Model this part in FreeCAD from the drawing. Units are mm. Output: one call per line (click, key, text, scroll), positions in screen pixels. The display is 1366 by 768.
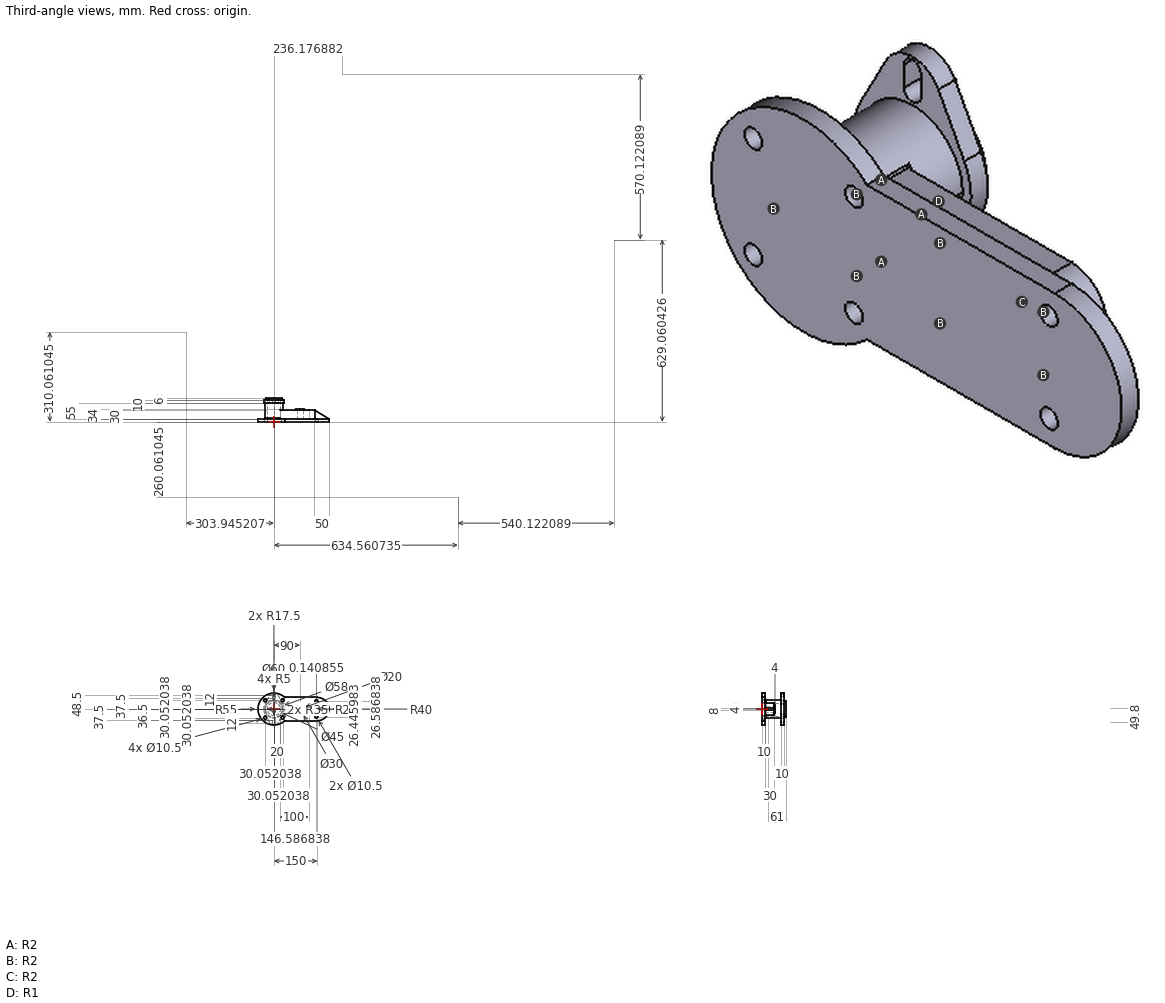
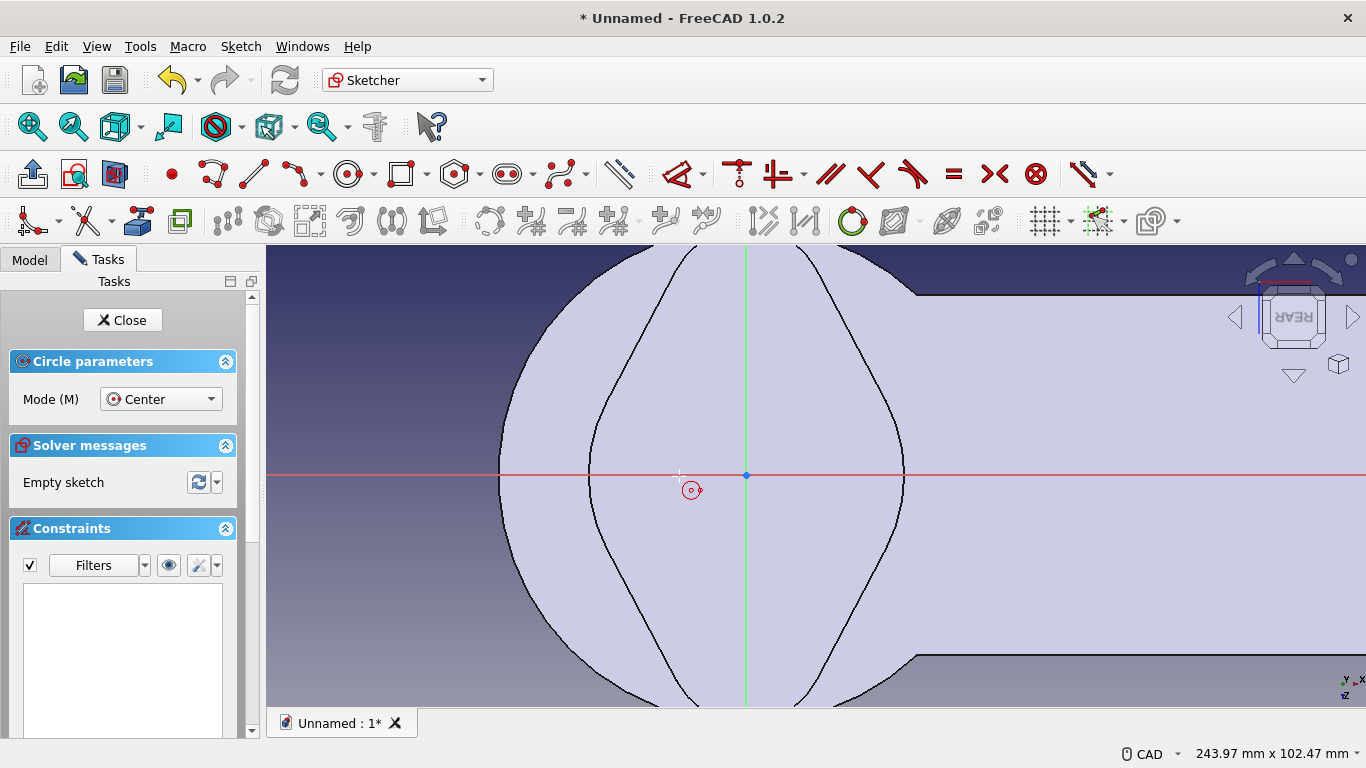
click(746, 475)
click(839, 383)
key(Escape)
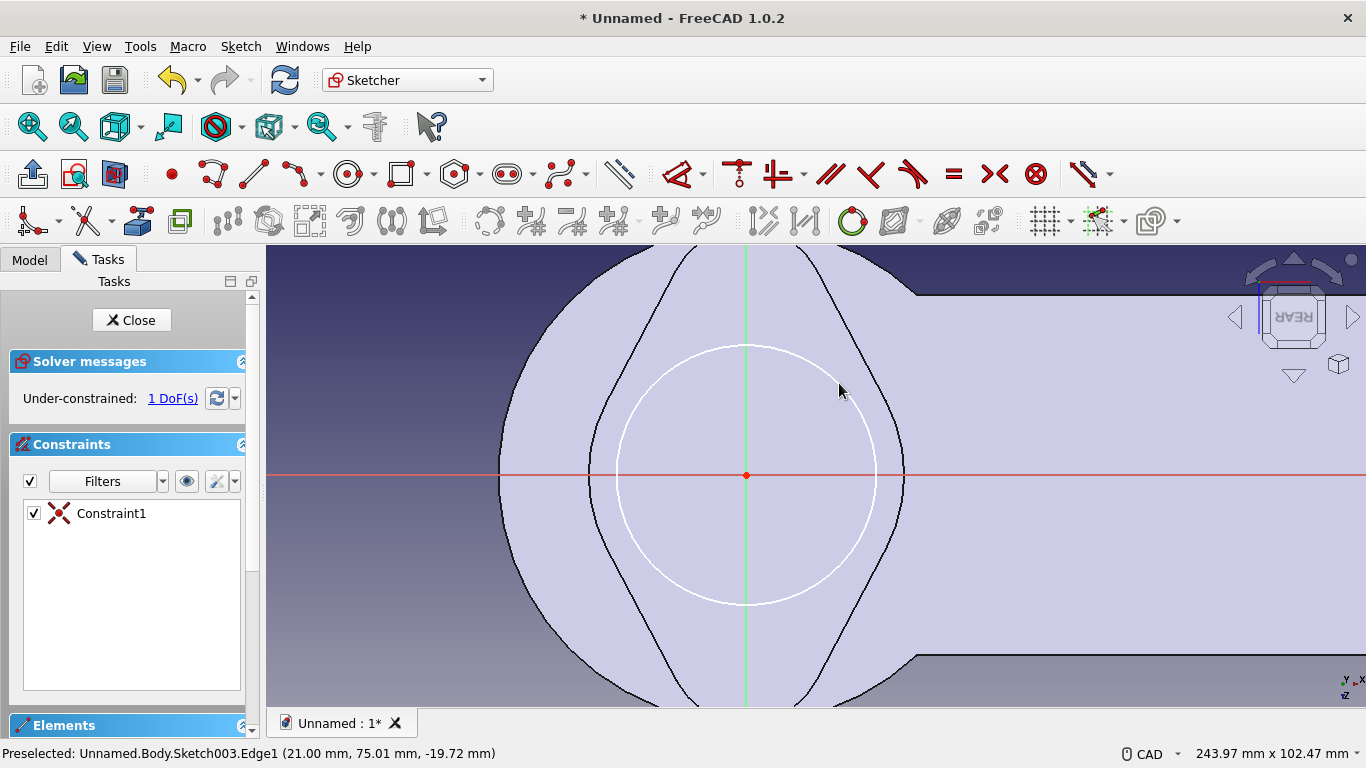
key(d)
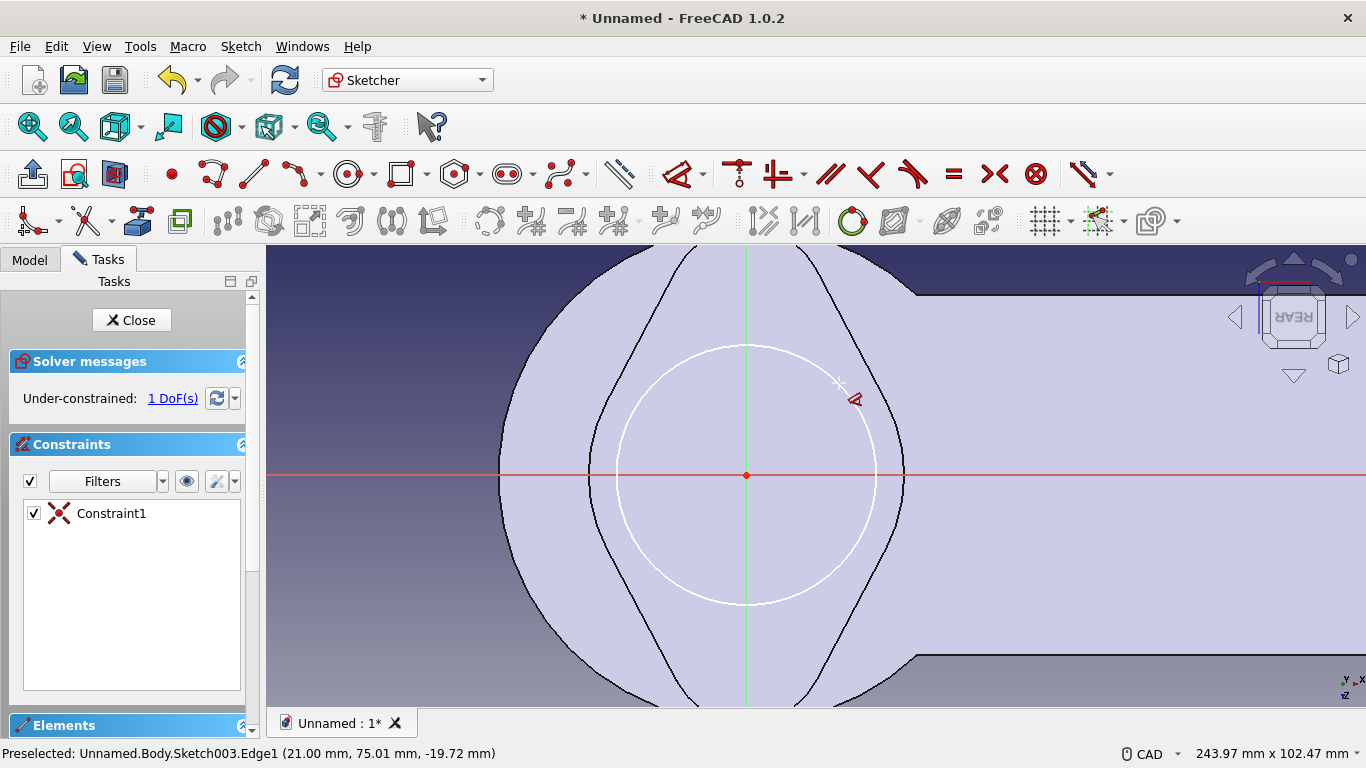
click(838, 383)
click(861, 360)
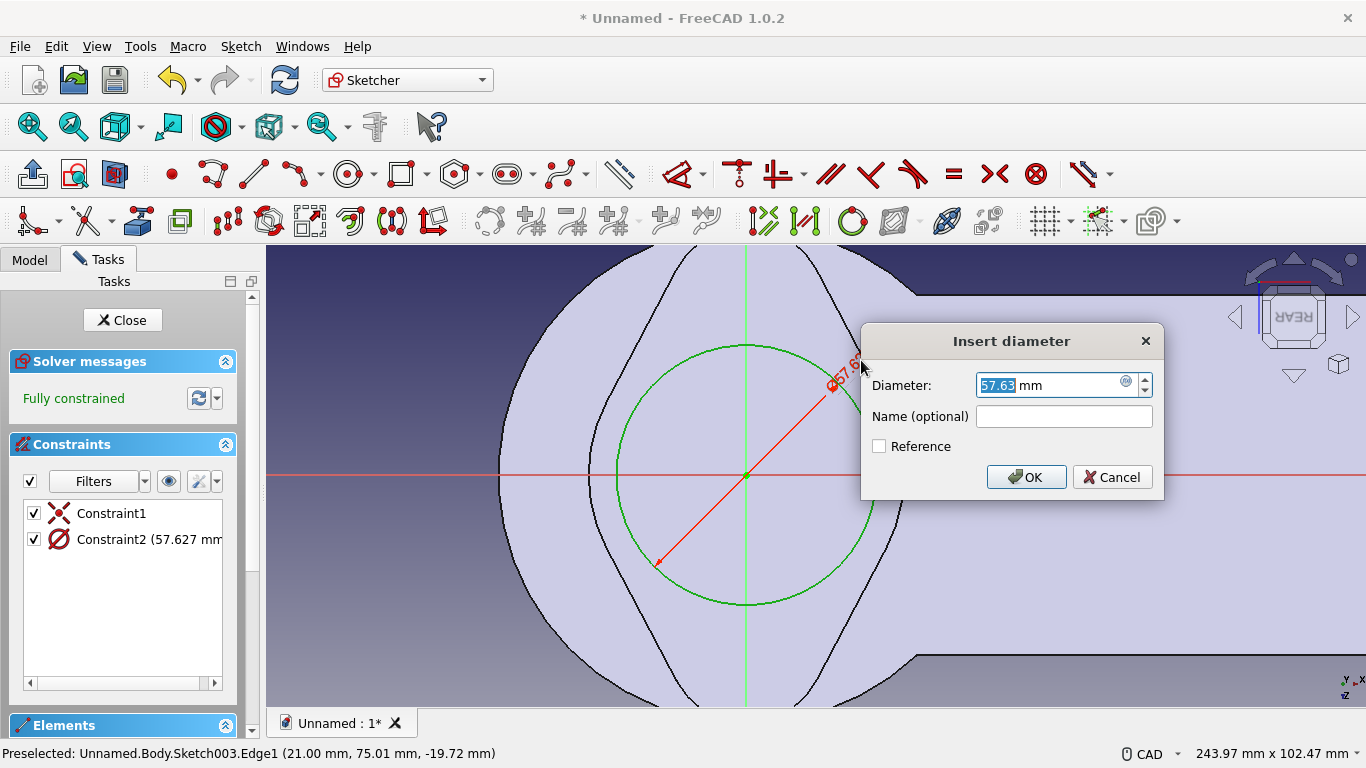
text(58)
key(Return)
key(Escape)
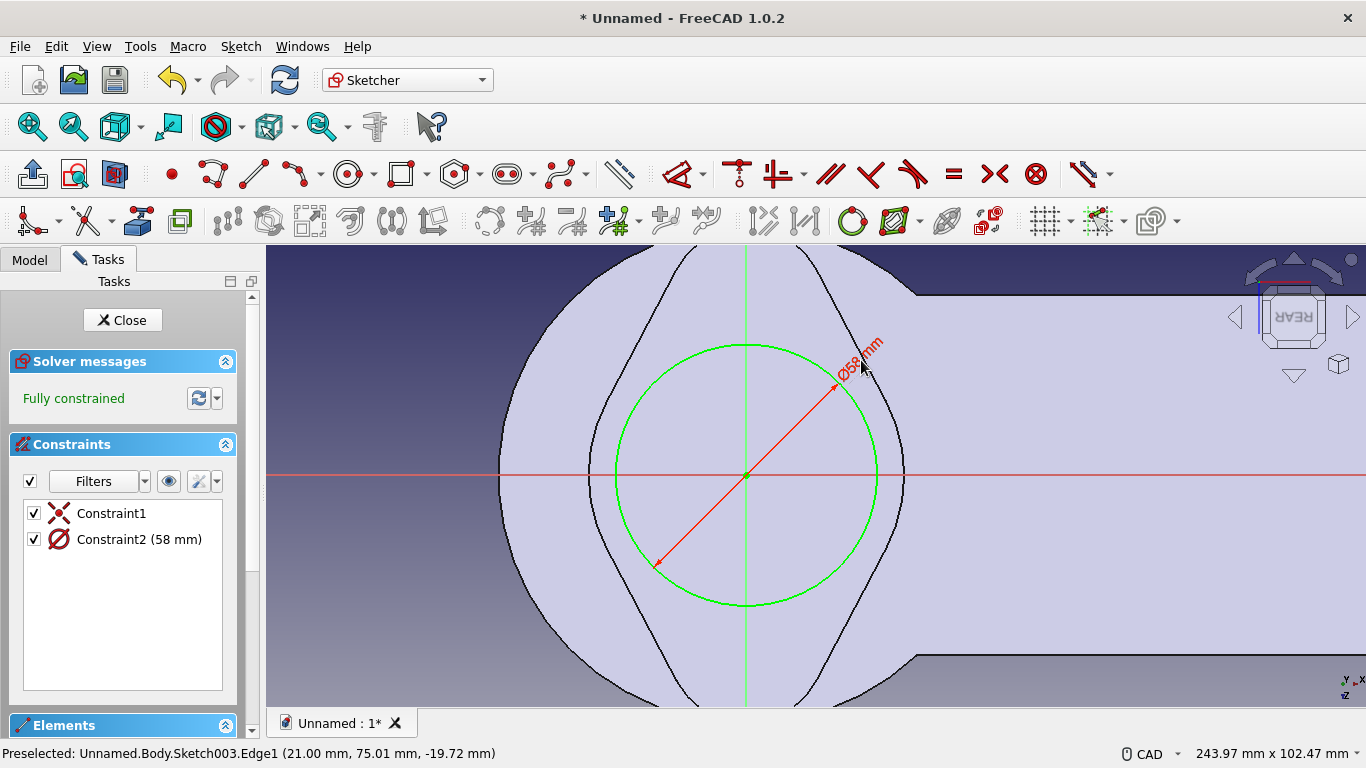
click(123, 320)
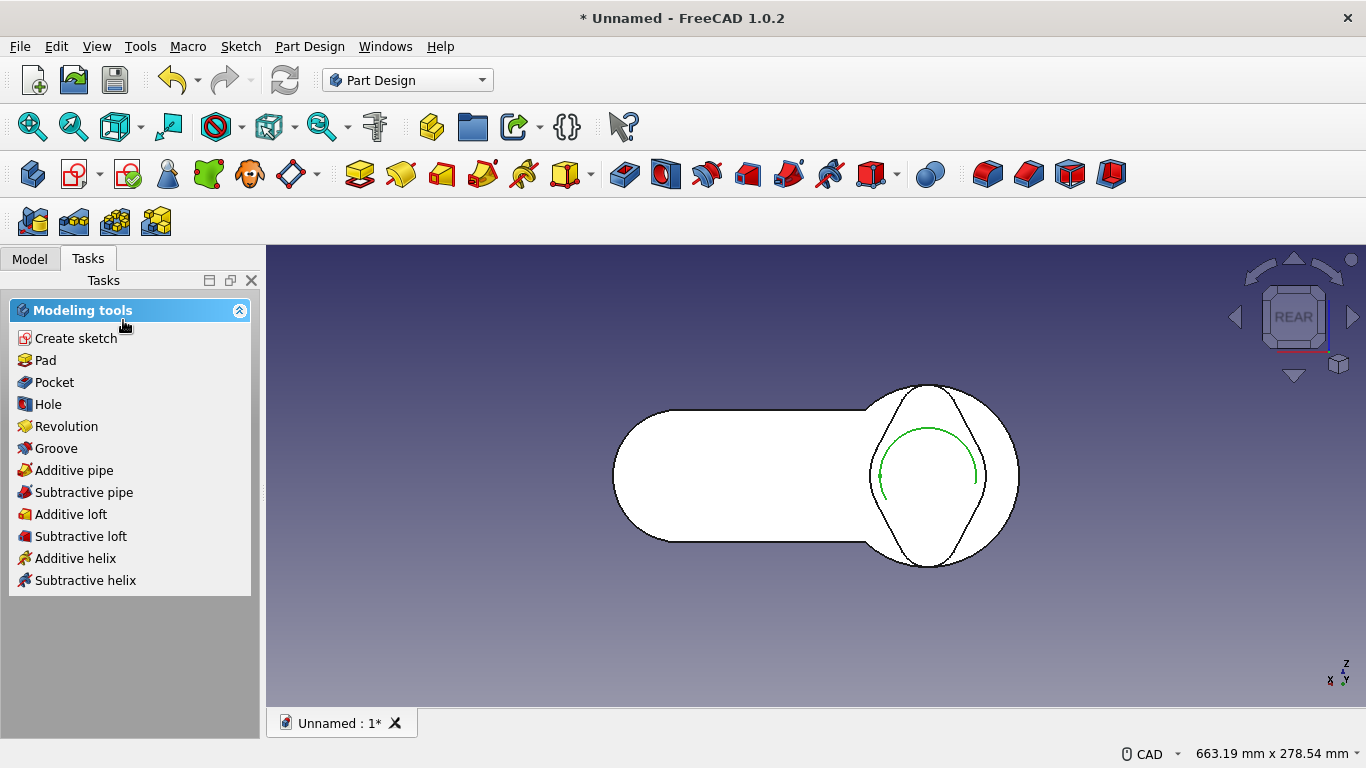
click(360, 174)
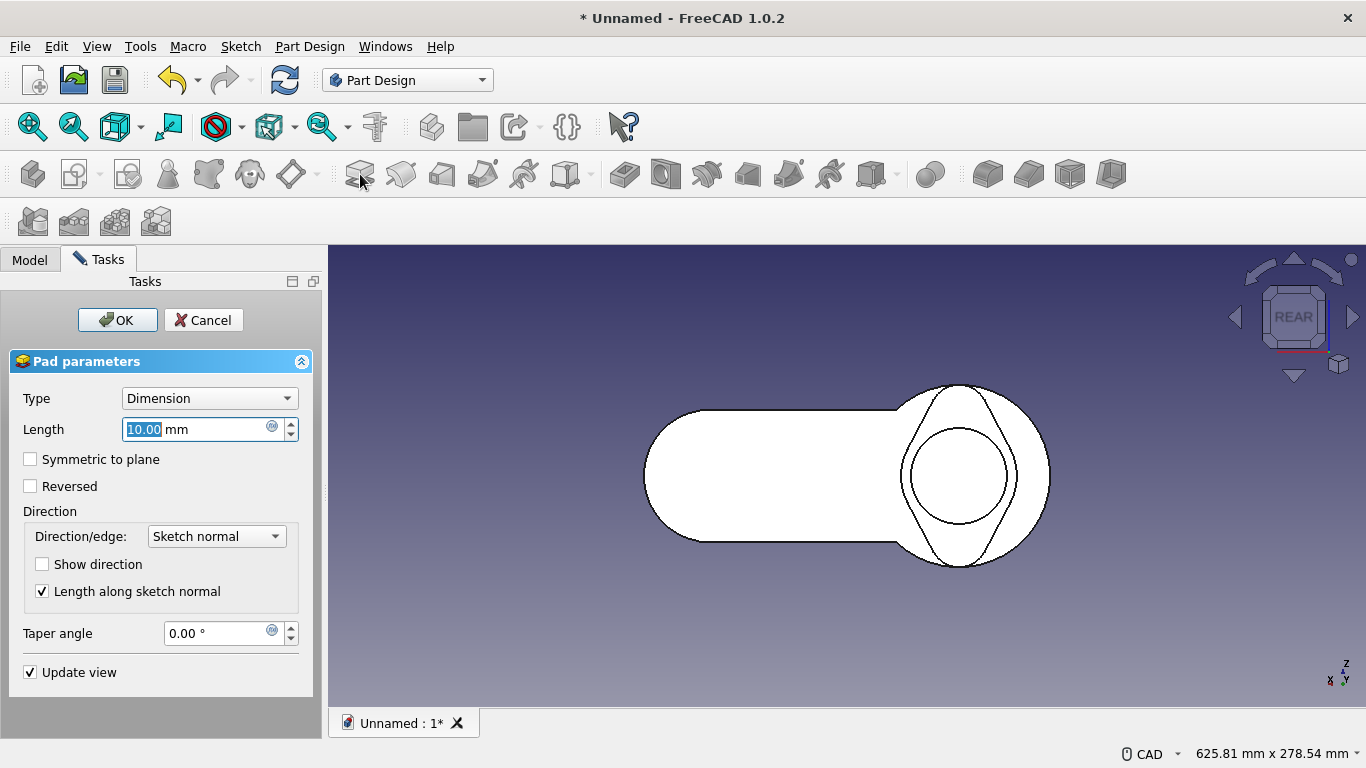
text(6)
key(Tab)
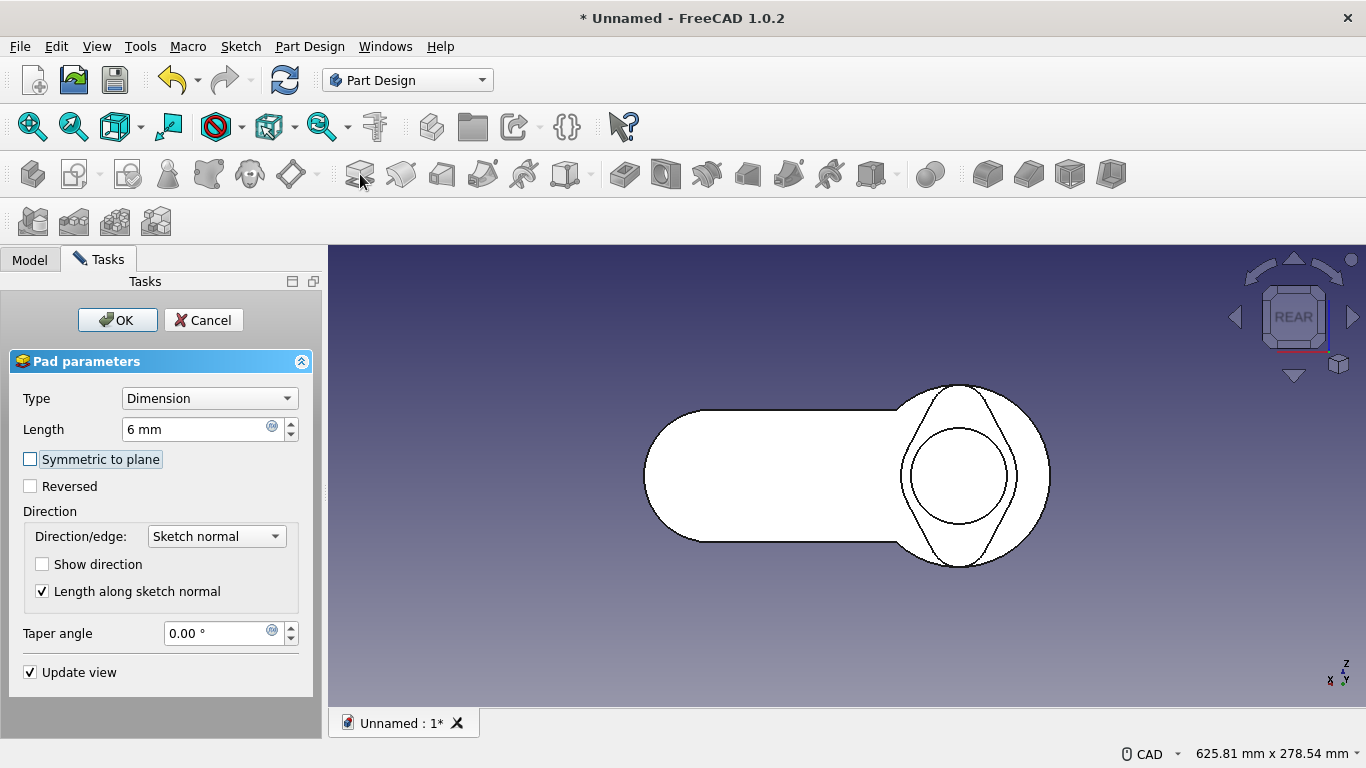
click(118, 320)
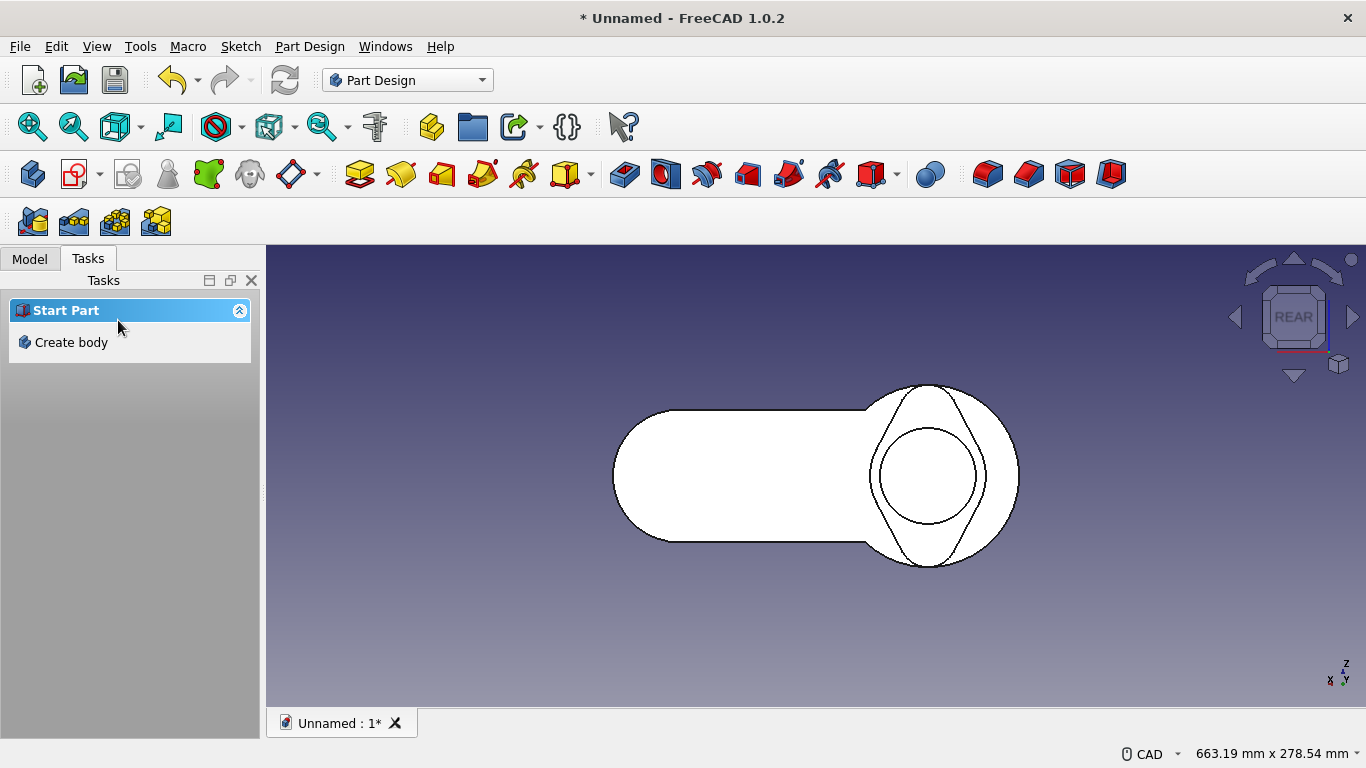
key(v)
key(f)